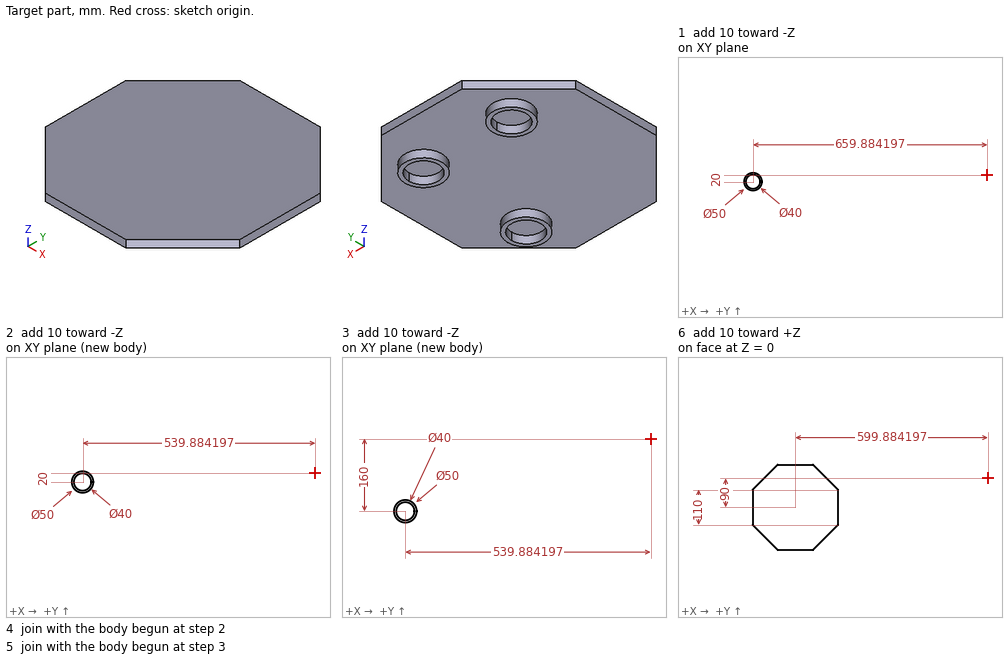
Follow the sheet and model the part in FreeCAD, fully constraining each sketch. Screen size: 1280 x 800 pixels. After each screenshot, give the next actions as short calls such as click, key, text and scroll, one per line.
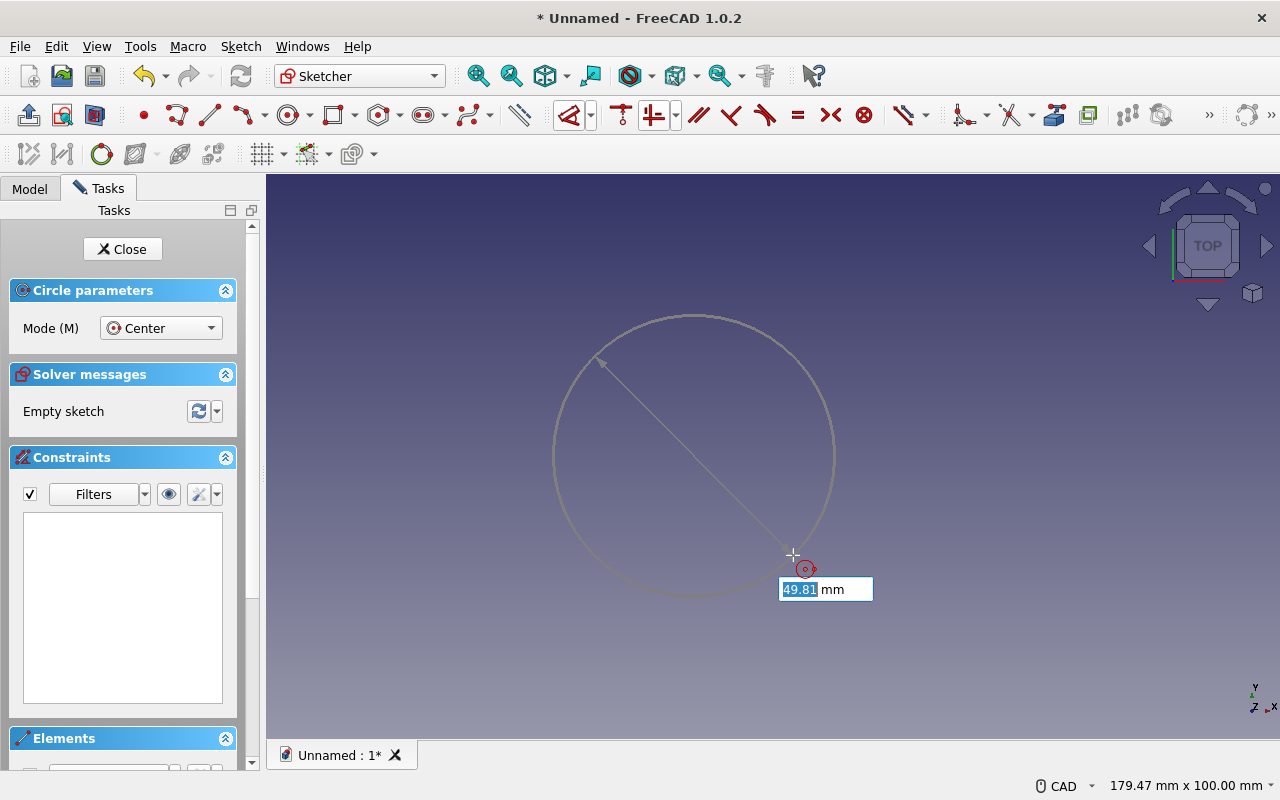
text(50)
key(Return)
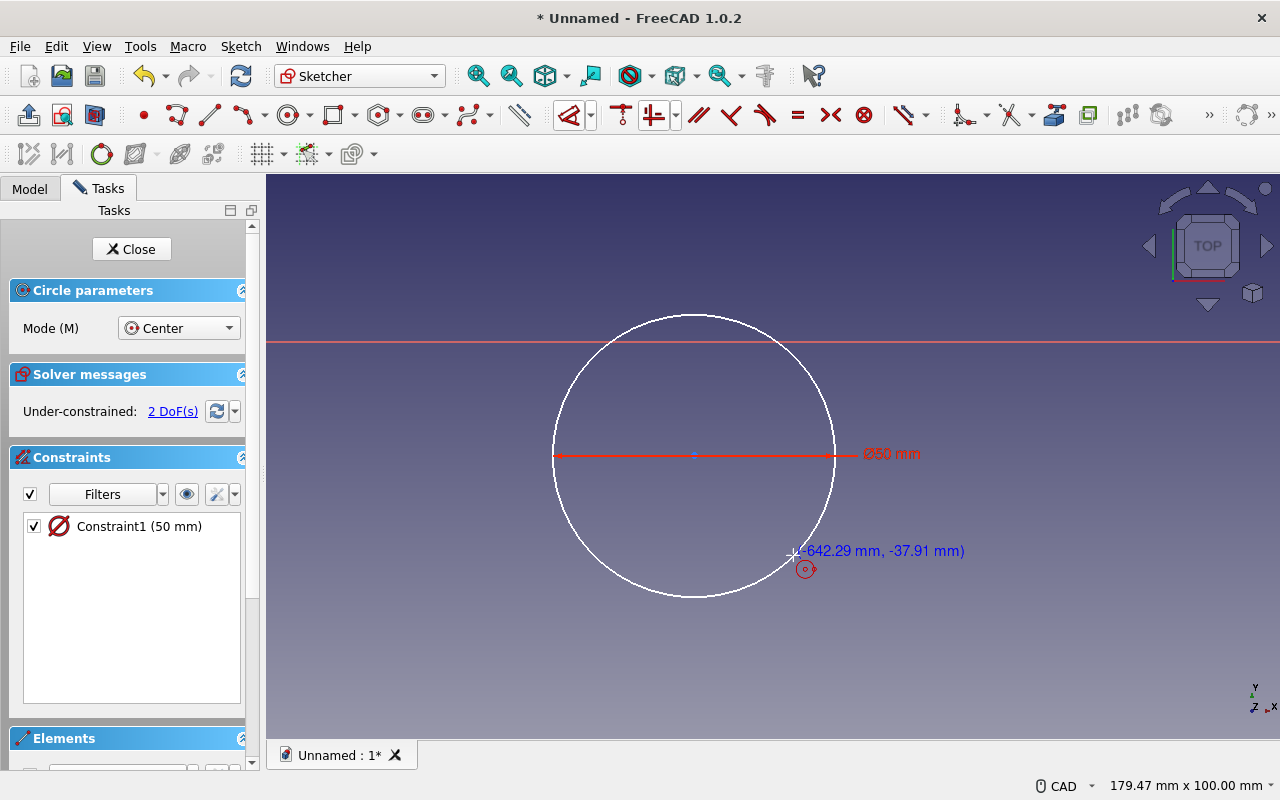
click(694, 456)
move(773, 375)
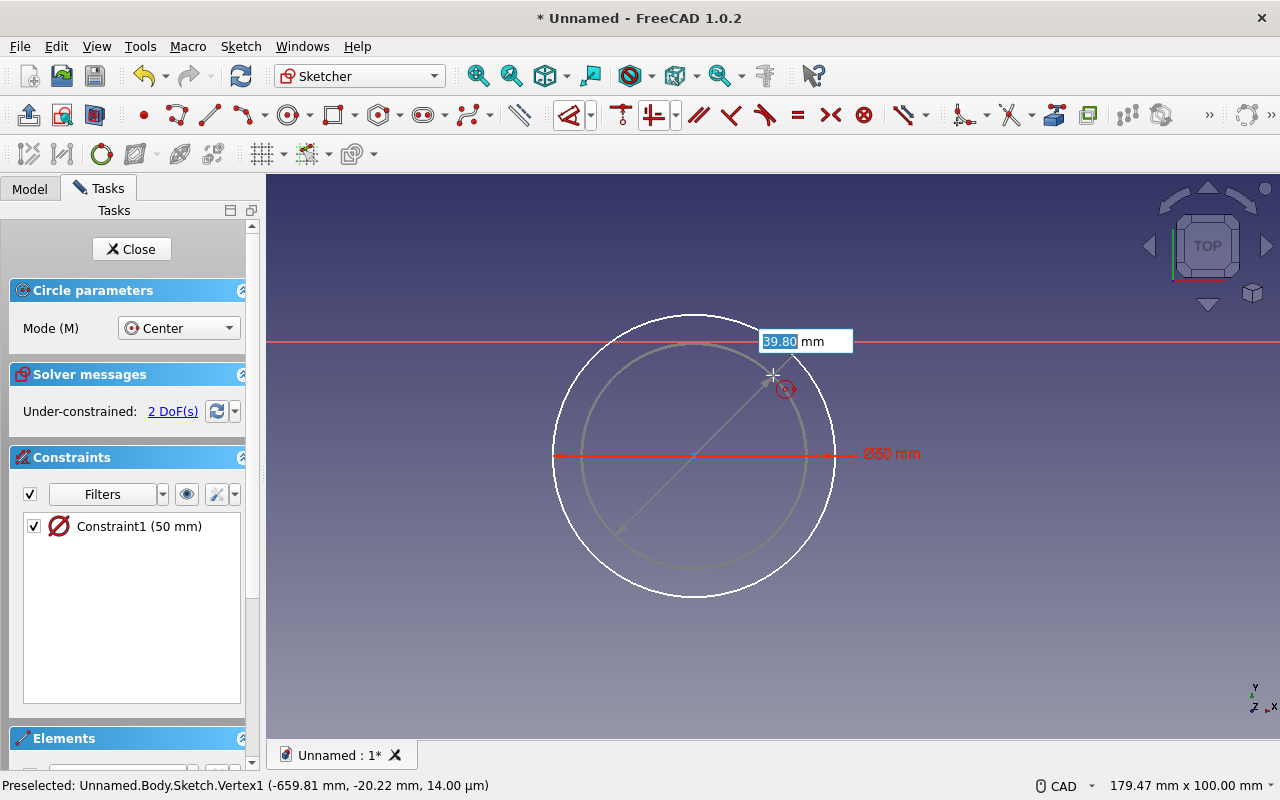
text(40)
key(Return)
key(Escape)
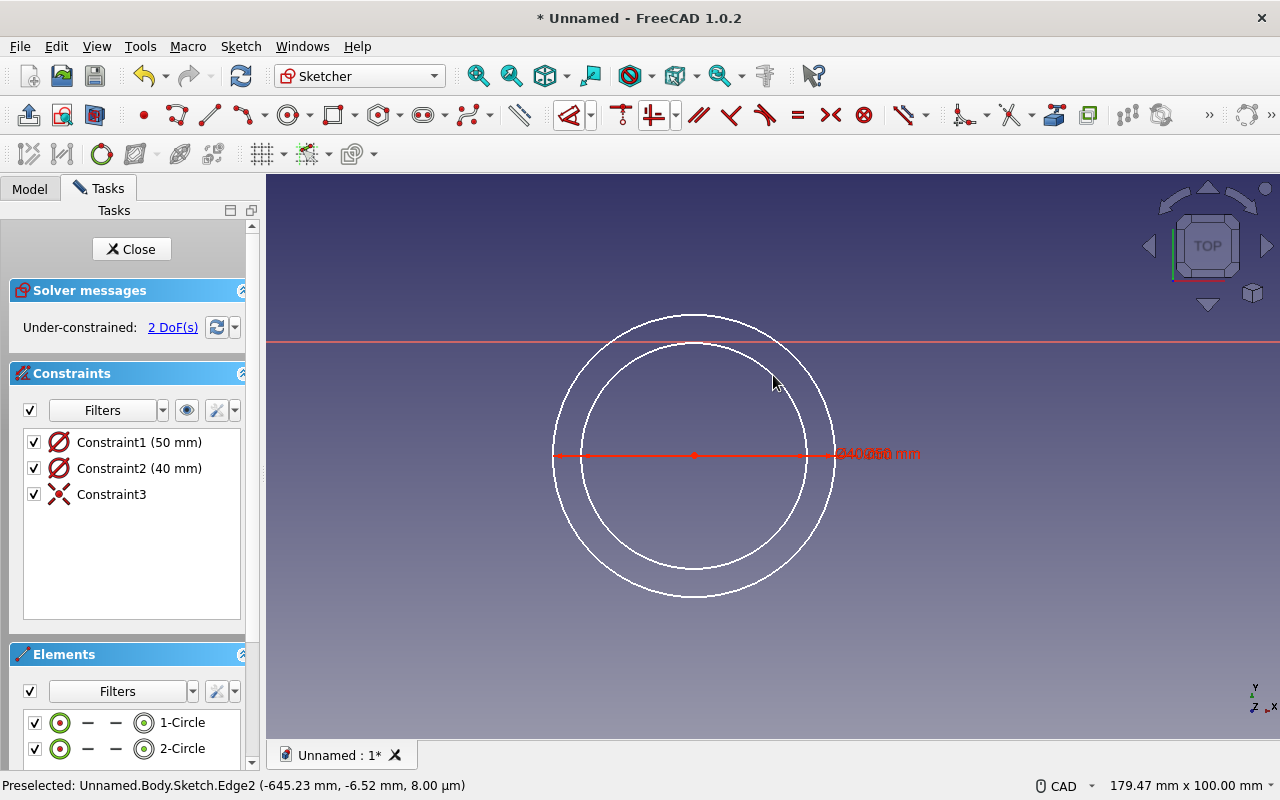
key(d)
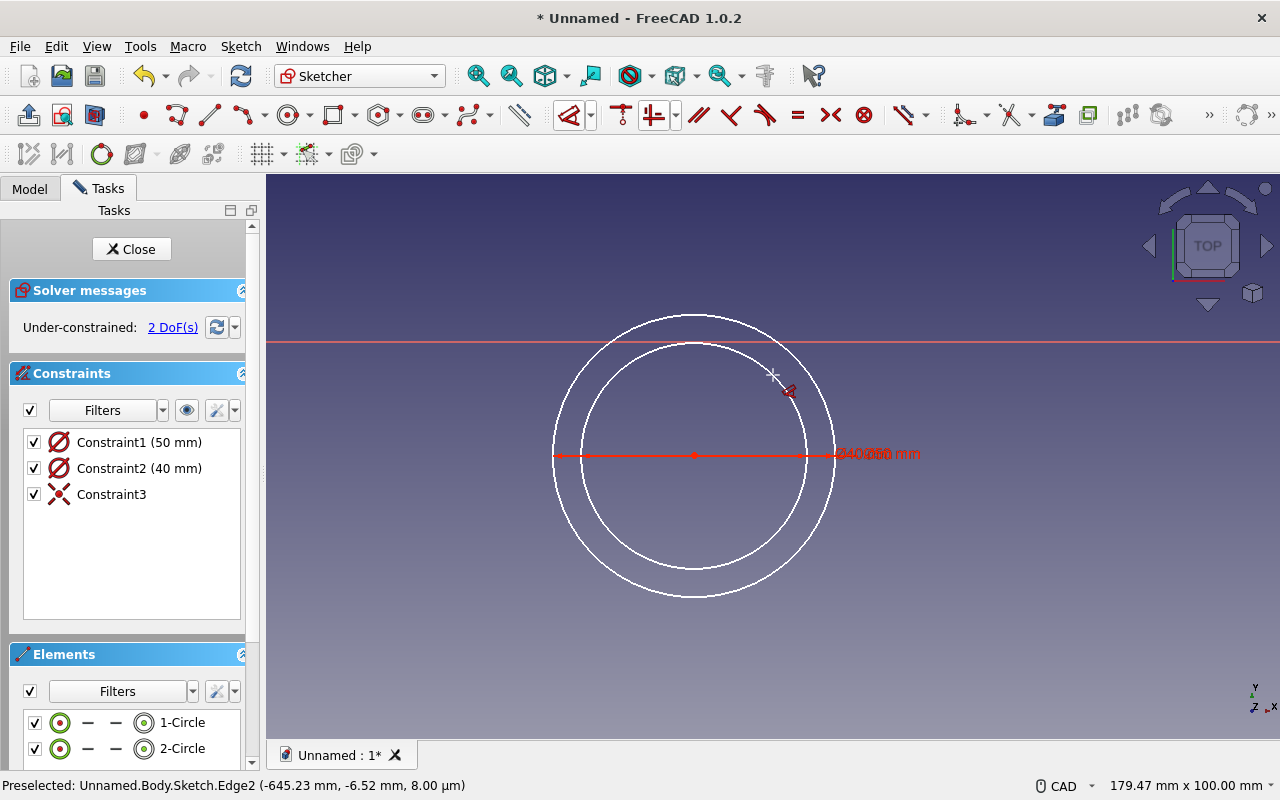
click(694, 456)
click(660, 399)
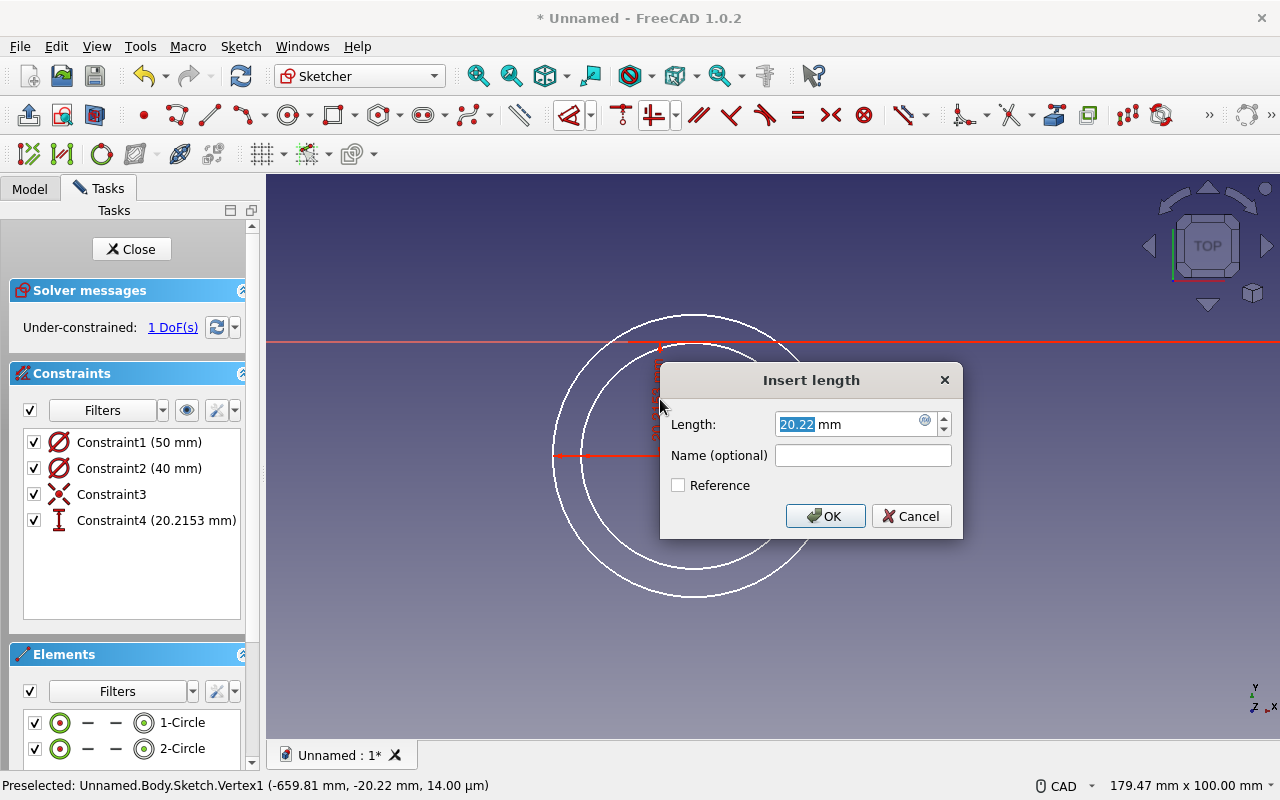
text(20)
key(Return)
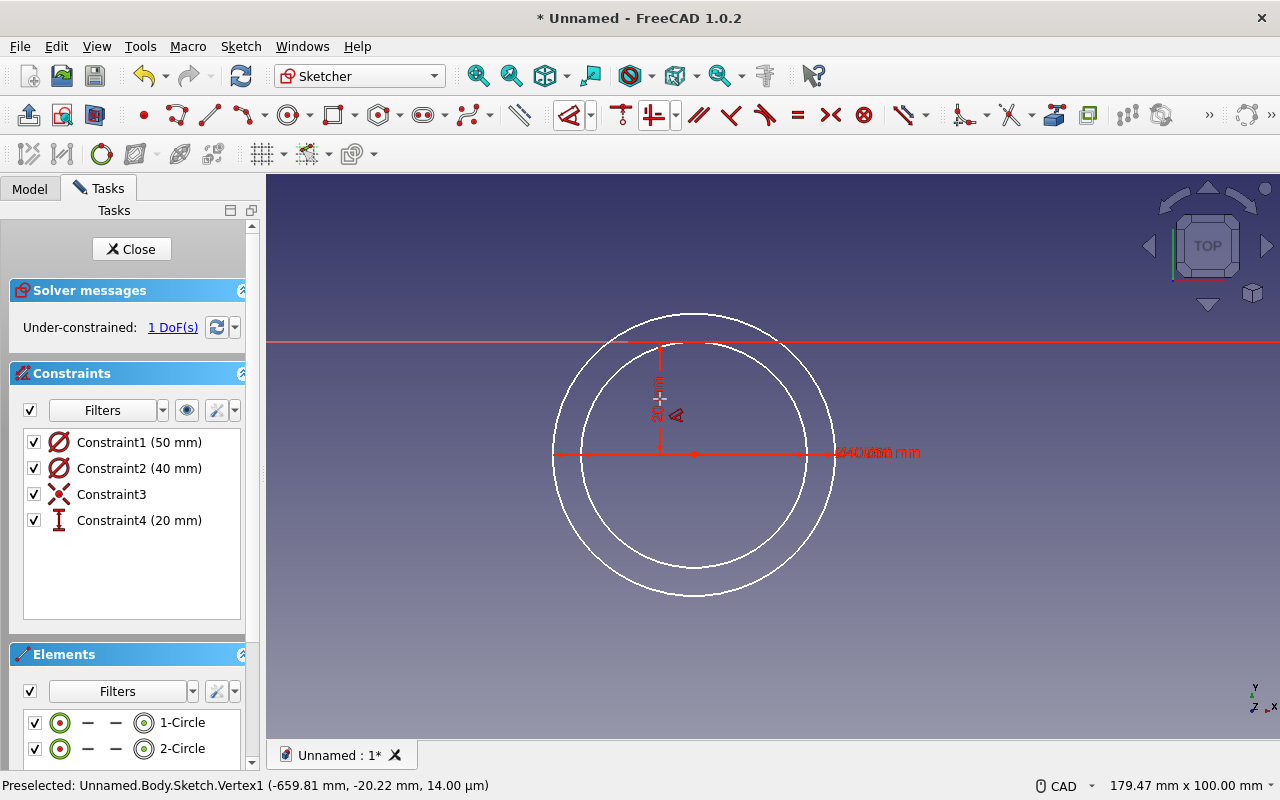
click(694, 455)
click(905, 308)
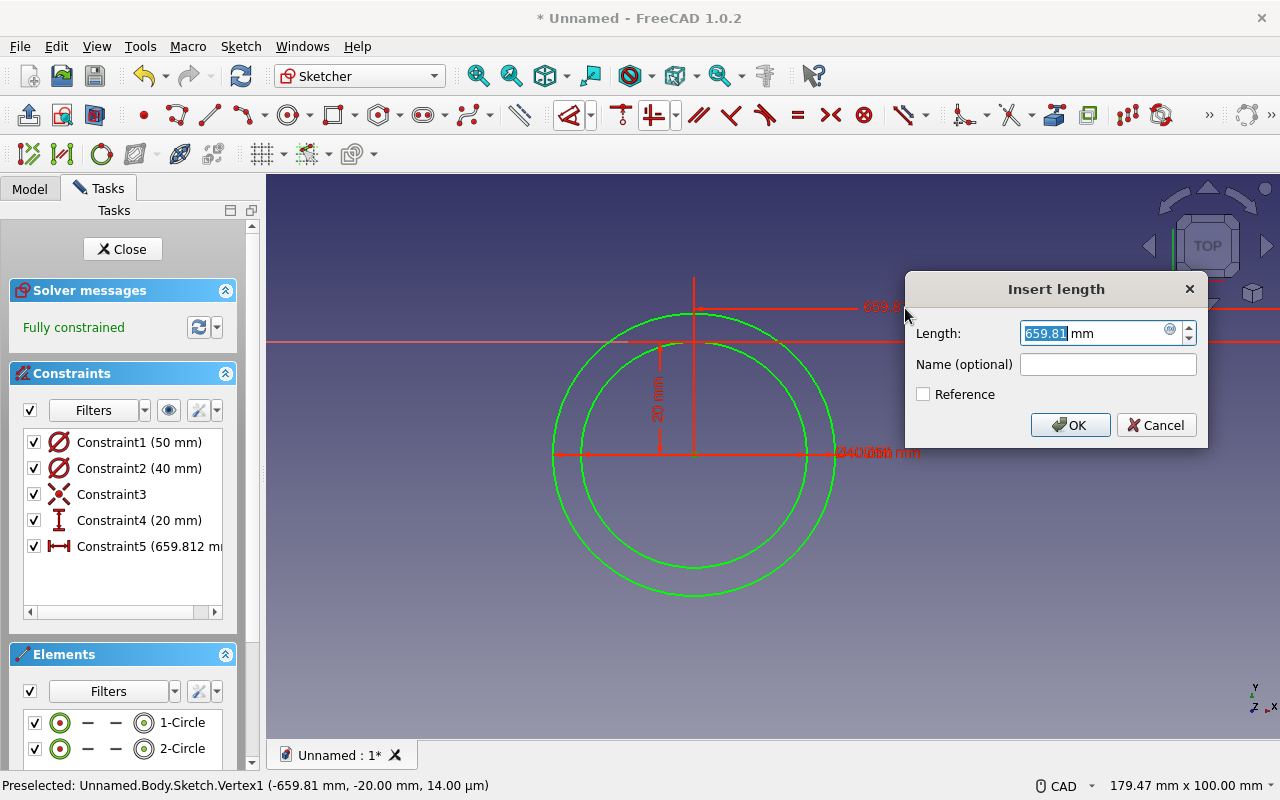
text(659.884197)
key(Return)
key(Escape)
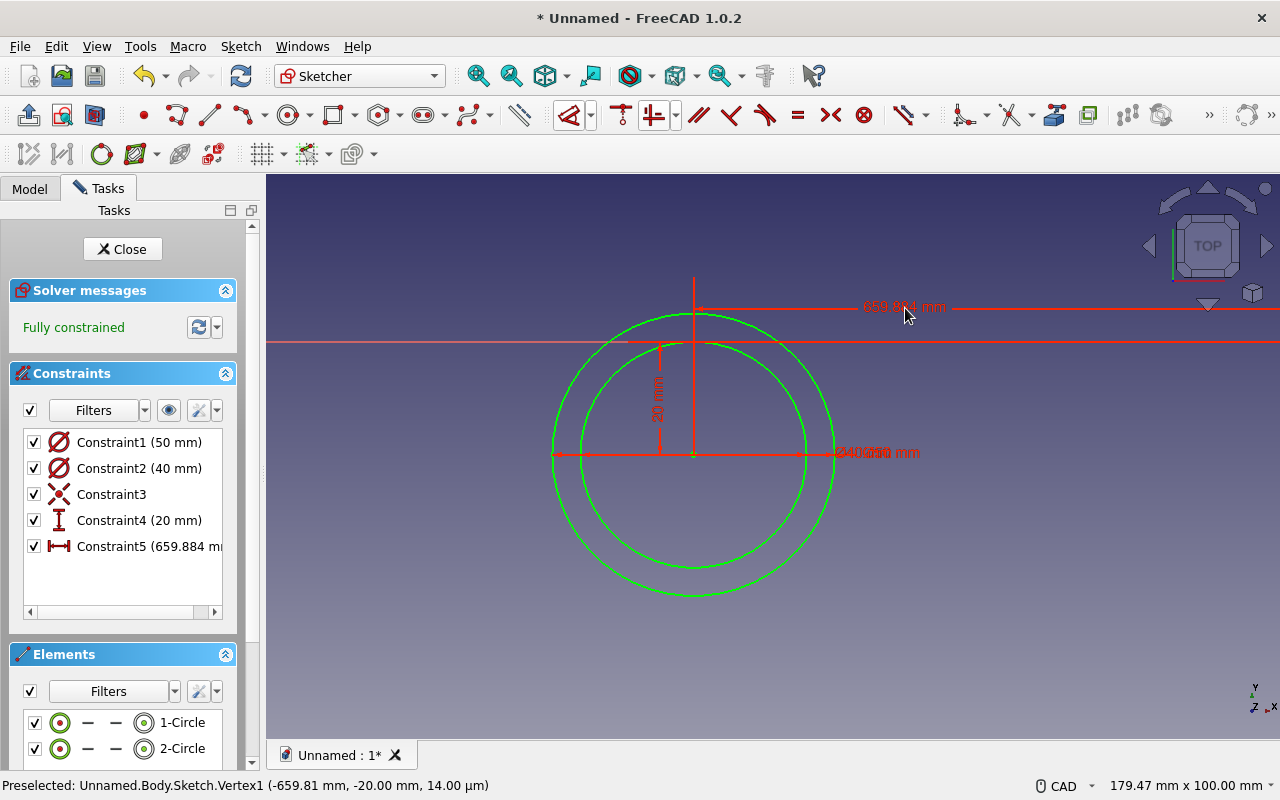
click(123, 249)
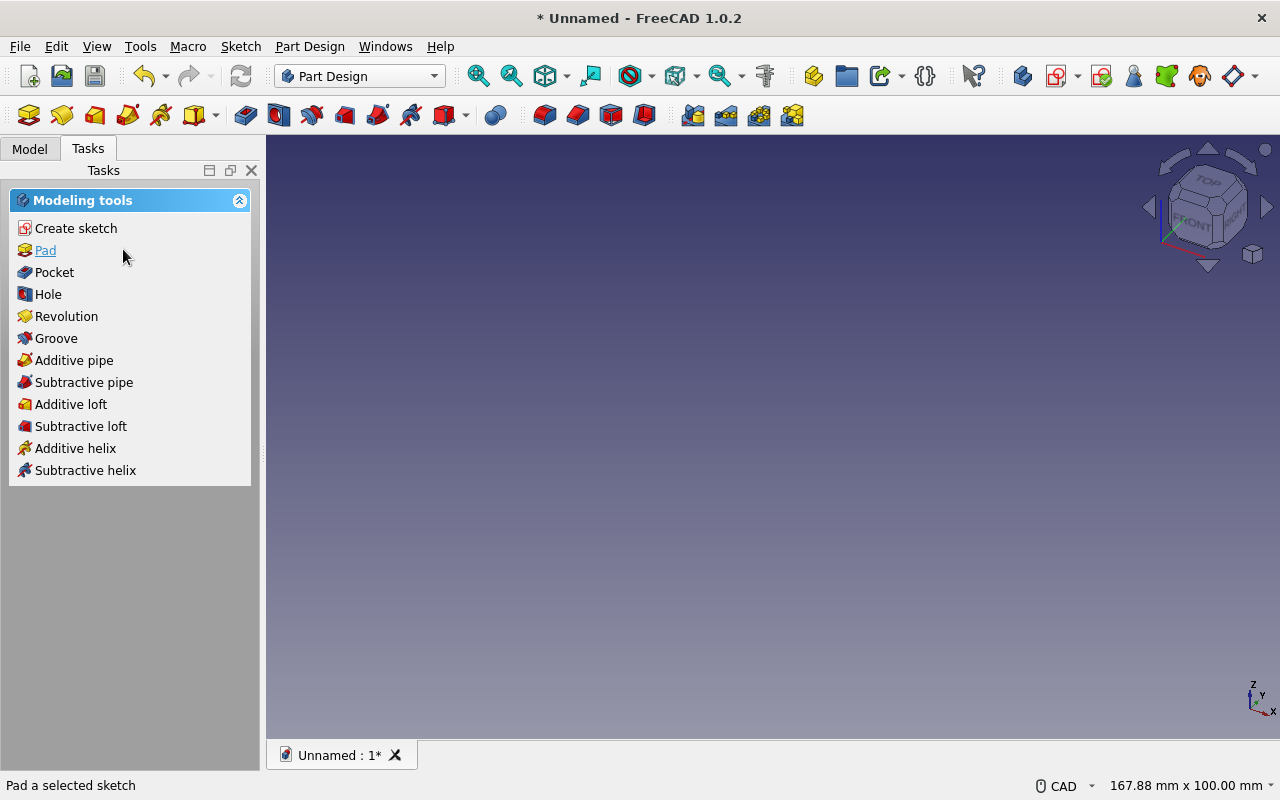
click(29, 116)